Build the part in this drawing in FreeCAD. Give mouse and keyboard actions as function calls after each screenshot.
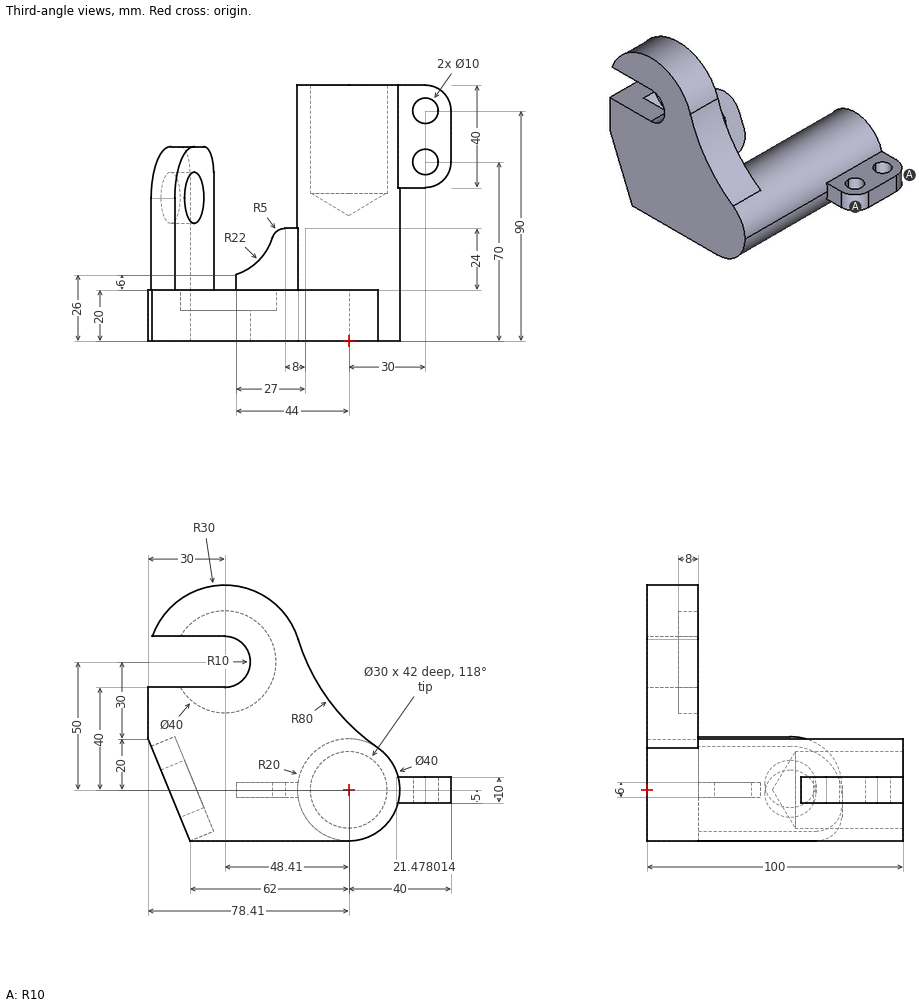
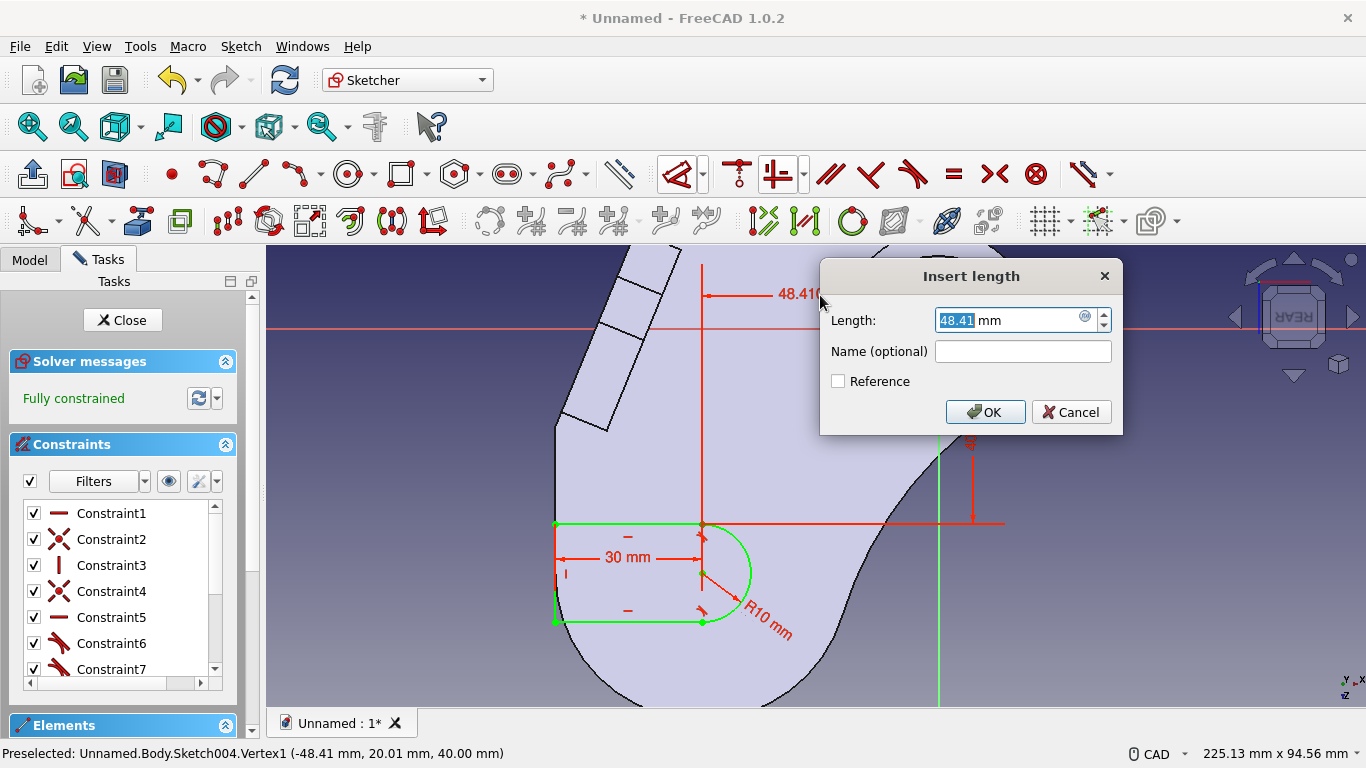
text(48.41)
key(Return)
key(Escape)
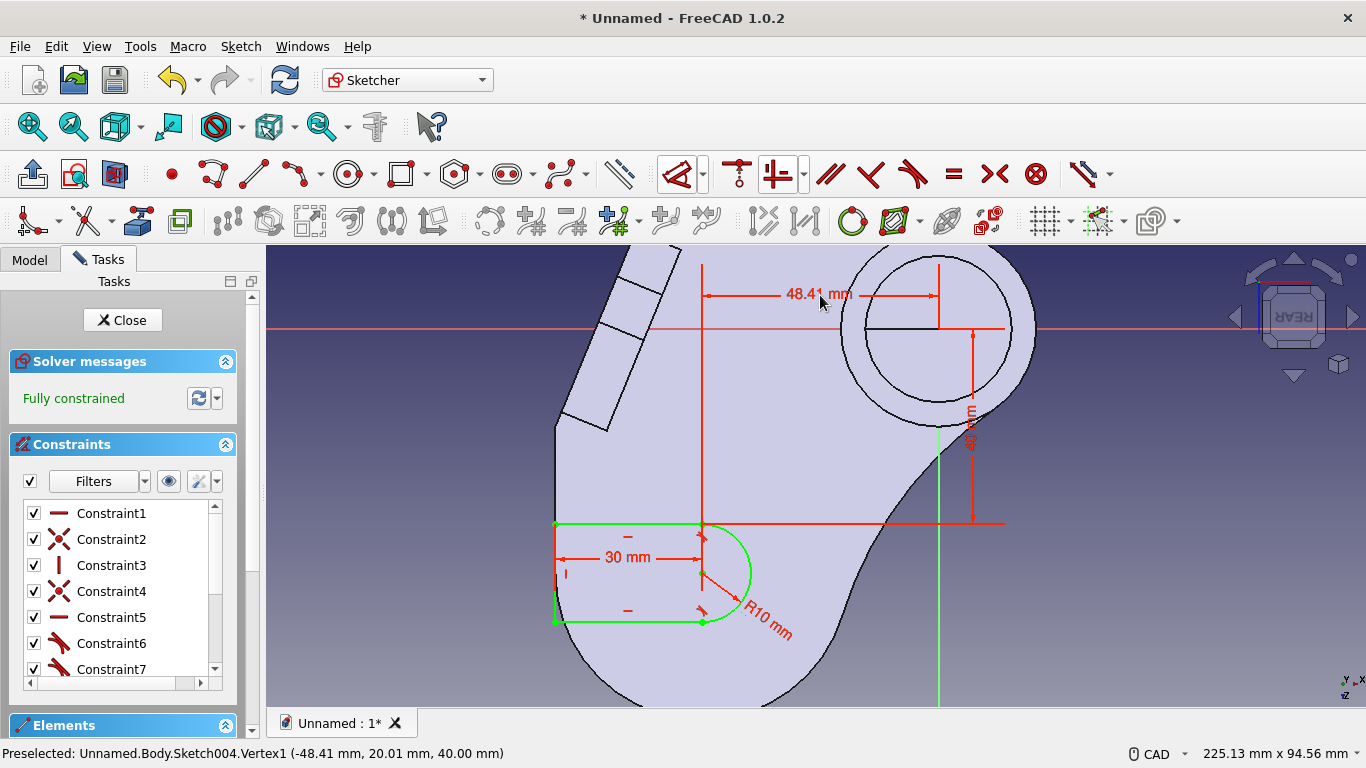
click(123, 320)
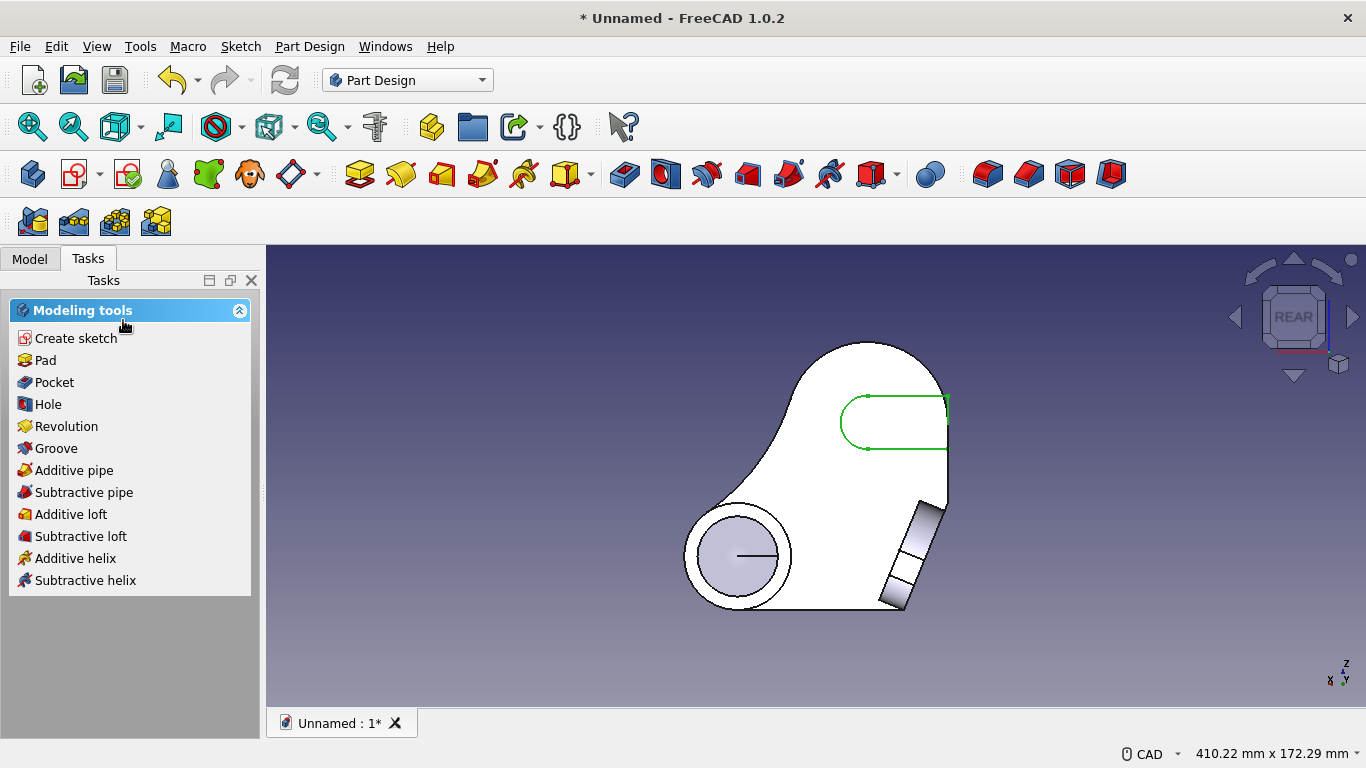
click(625, 174)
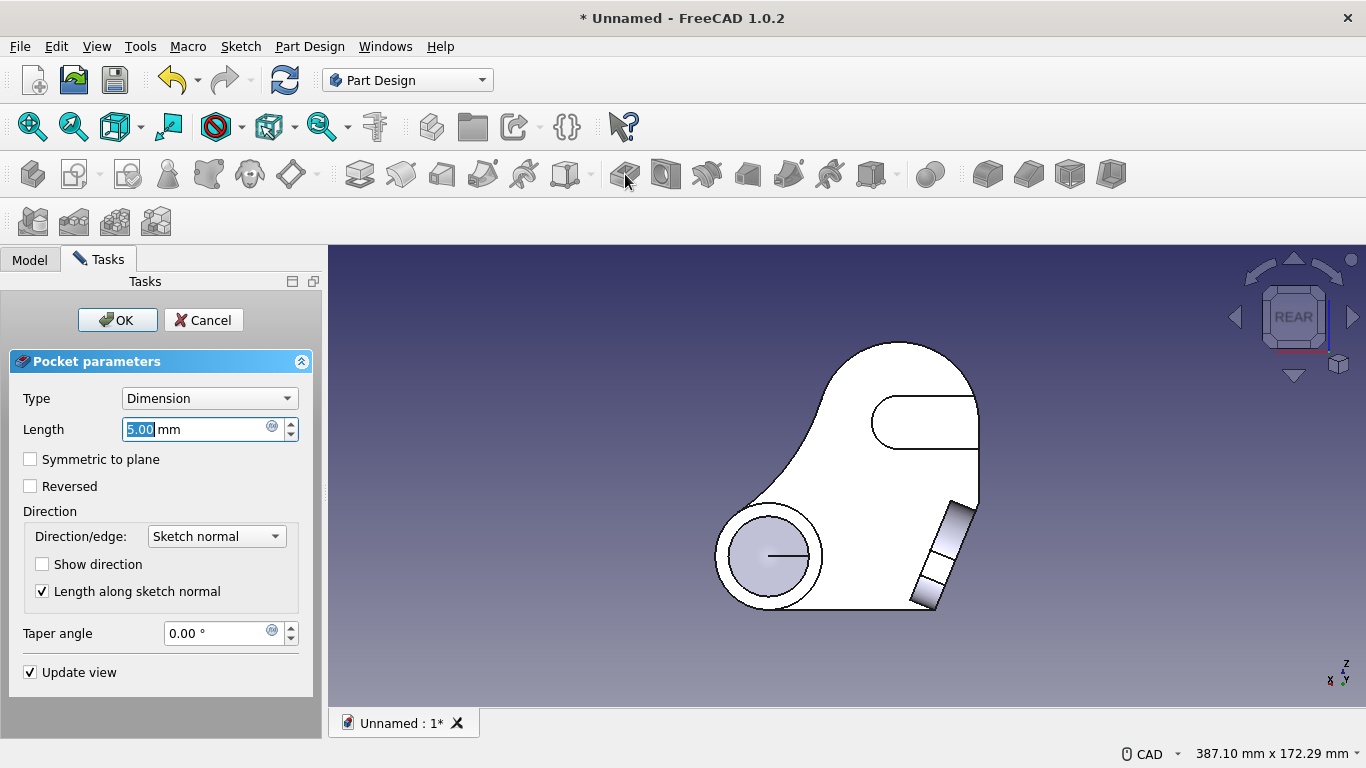
click(210, 398)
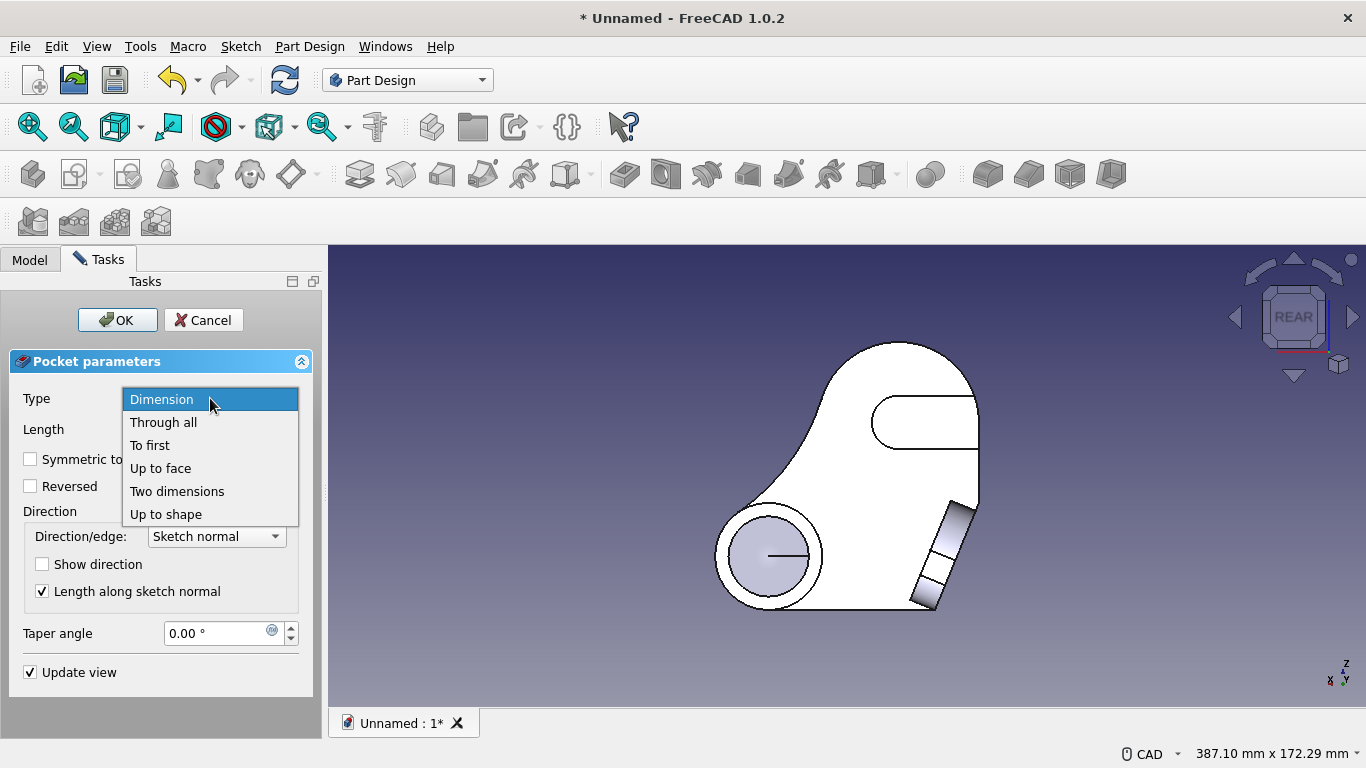
click(208, 422)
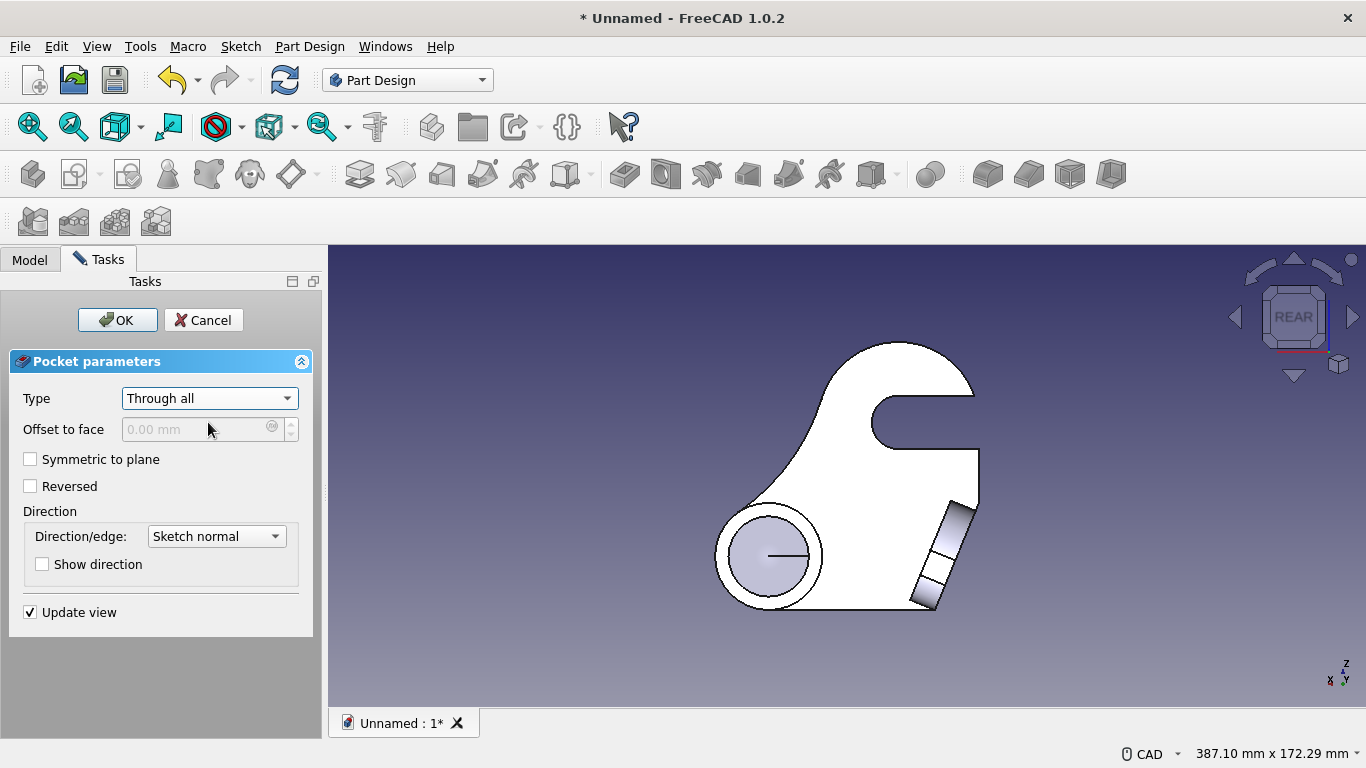
click(118, 320)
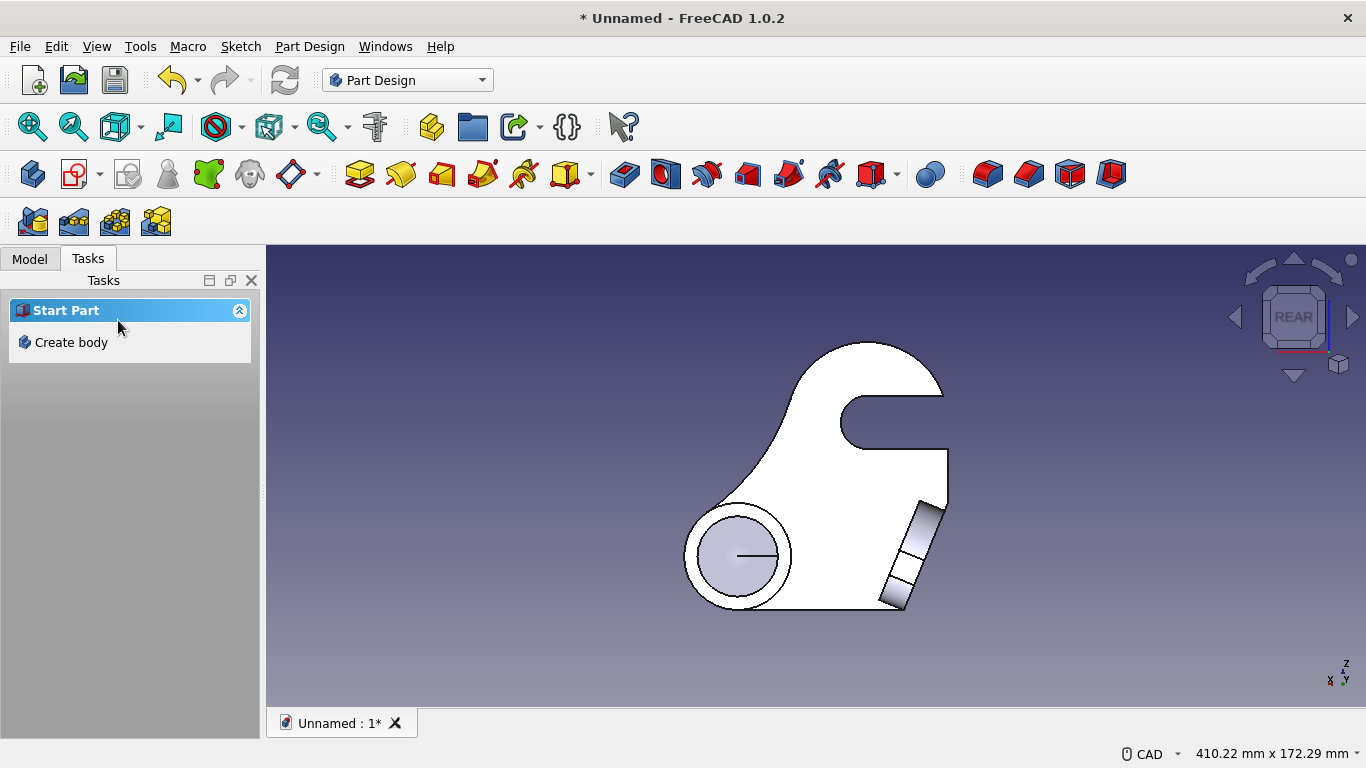
click(862, 513)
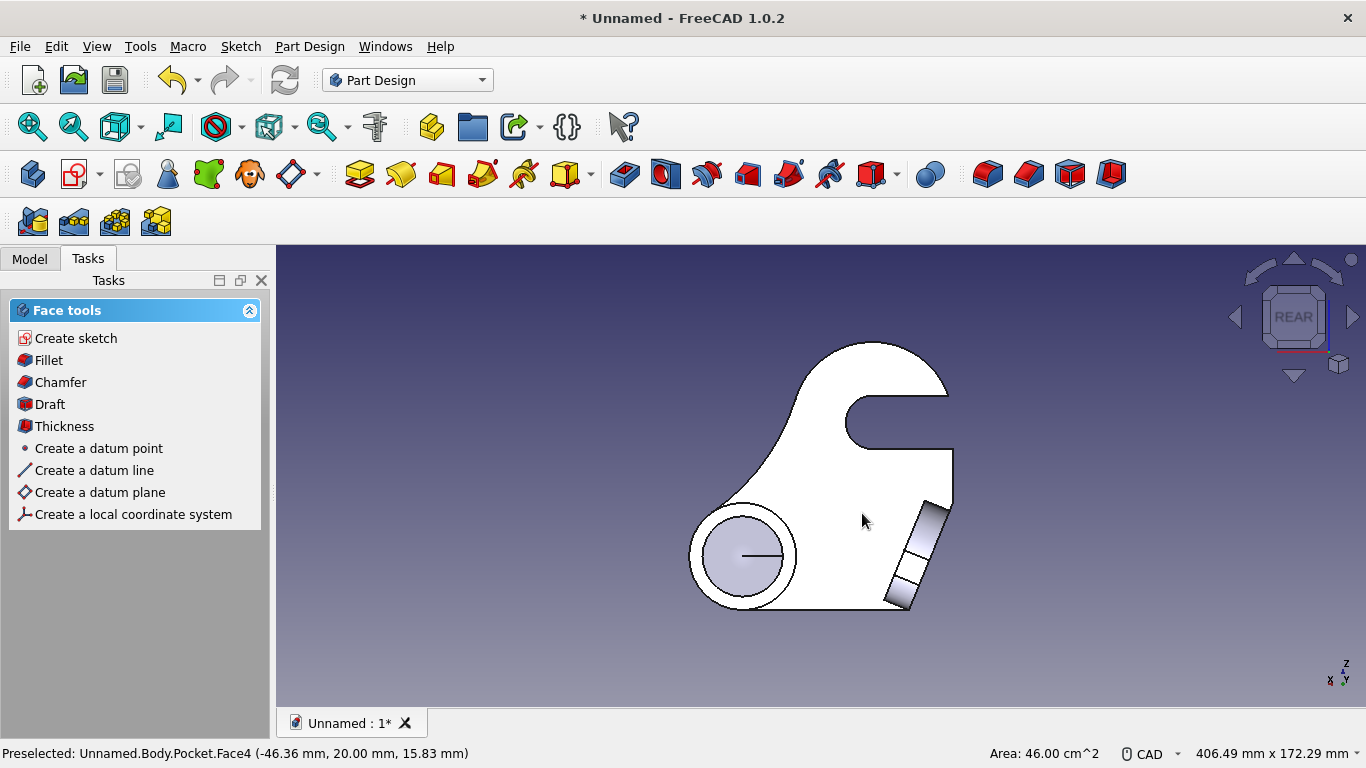
click(74, 174)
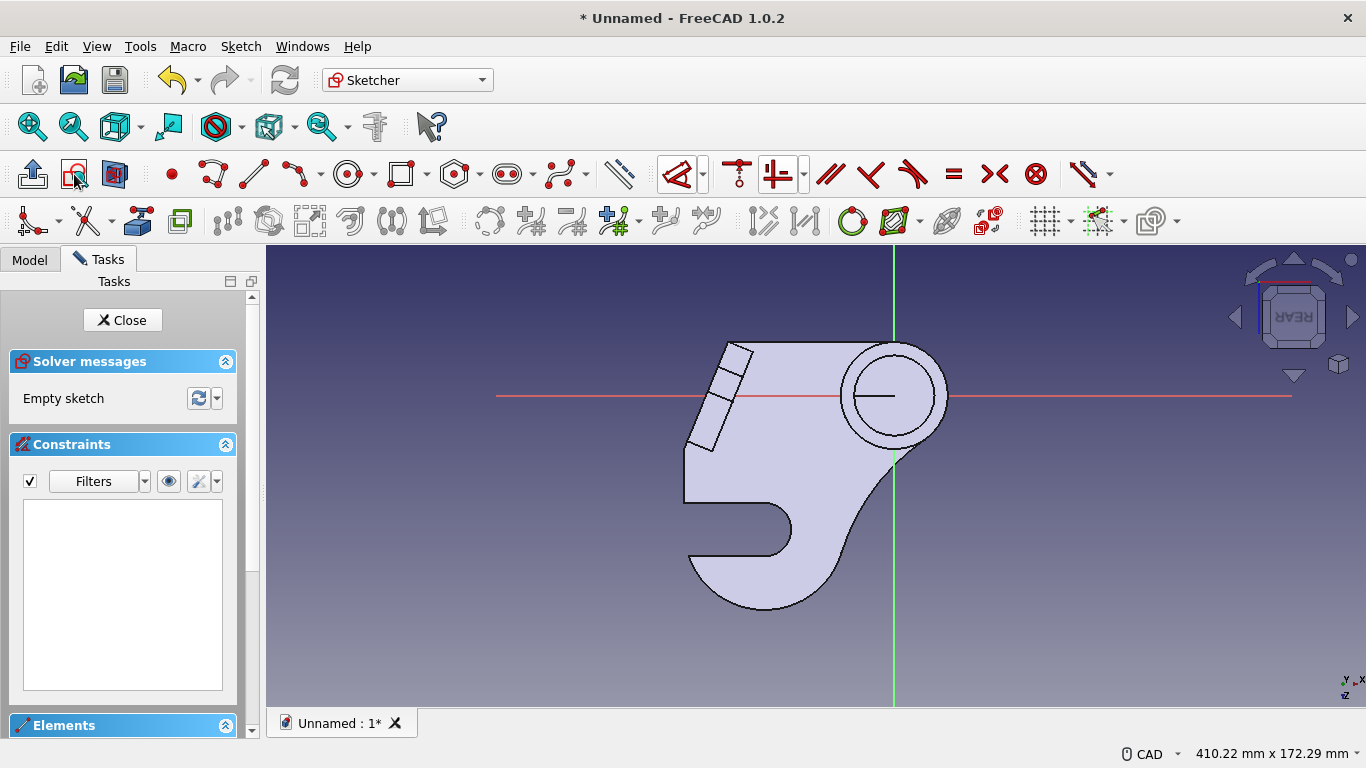
scroll(915, 517, up, 2)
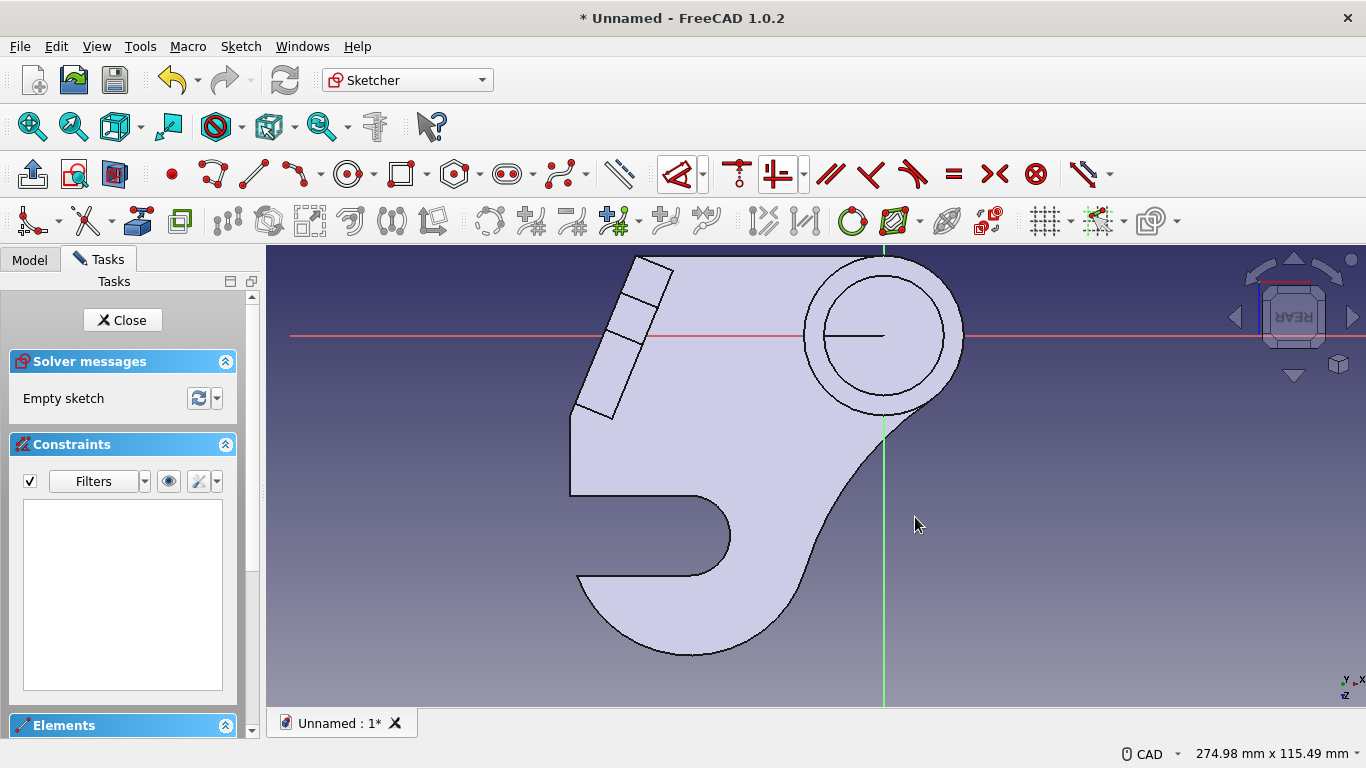
key(g)
key(c)